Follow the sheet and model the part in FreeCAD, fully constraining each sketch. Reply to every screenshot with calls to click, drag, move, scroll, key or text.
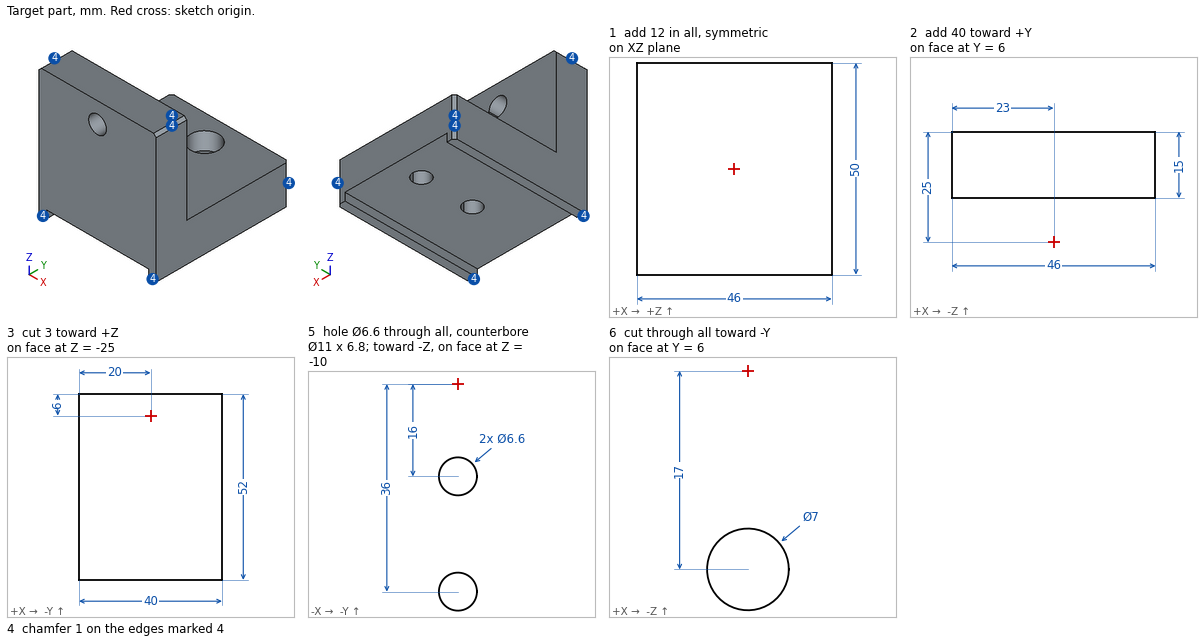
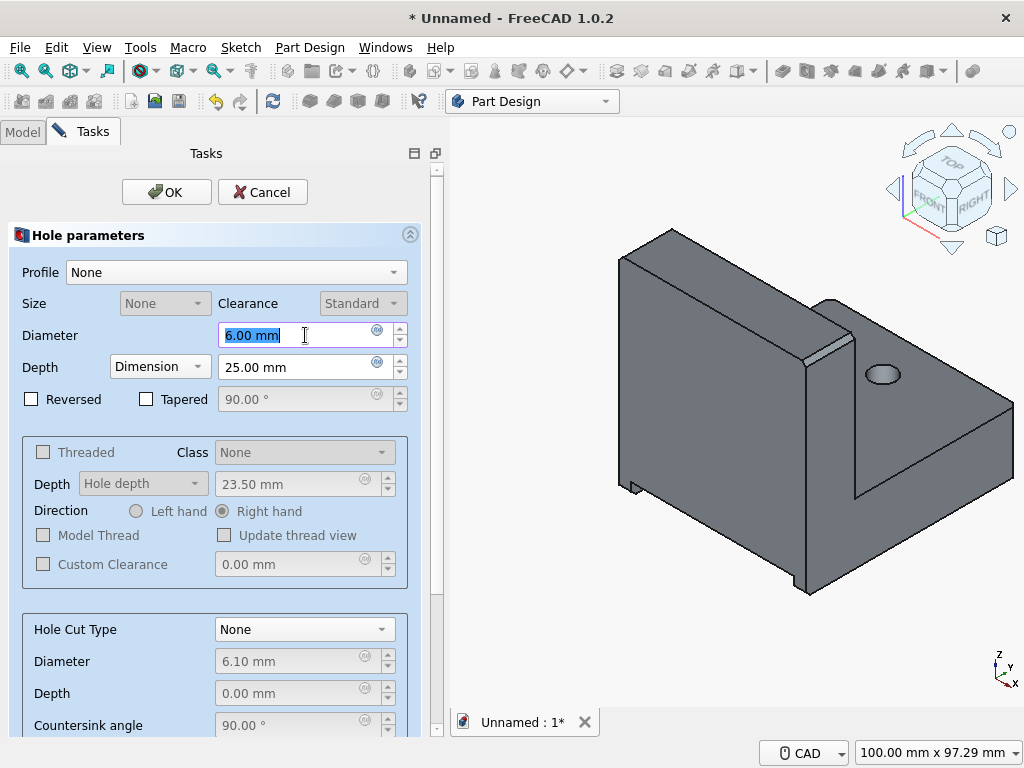
text(6.6)
key(Tab)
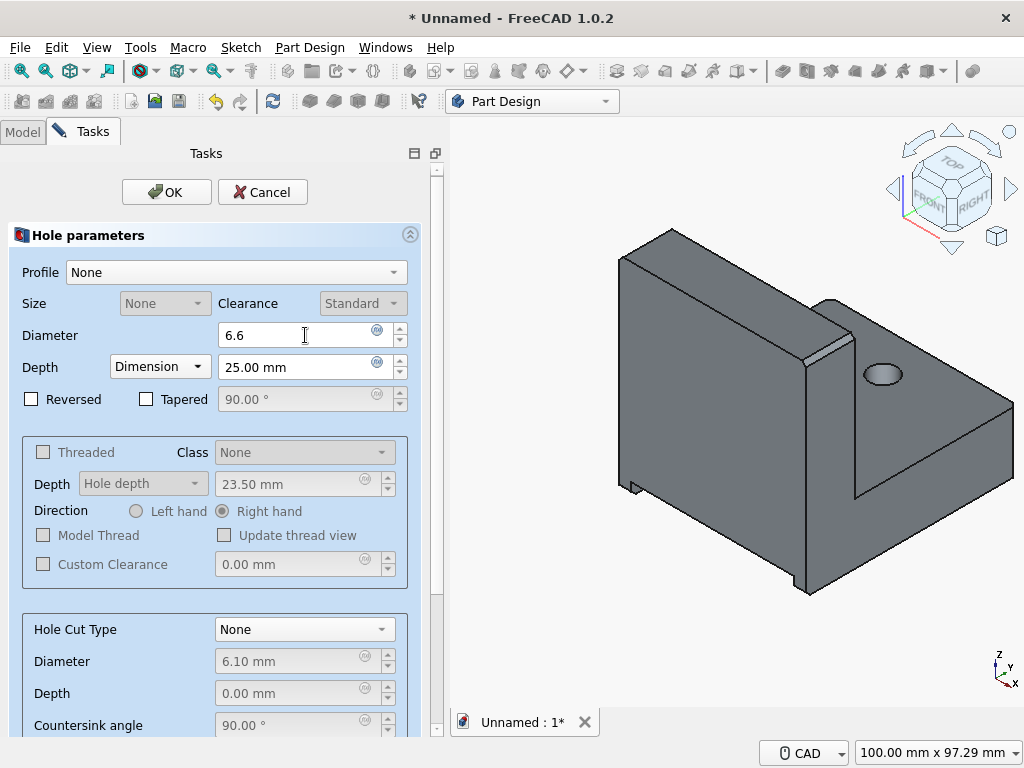
click(161, 366)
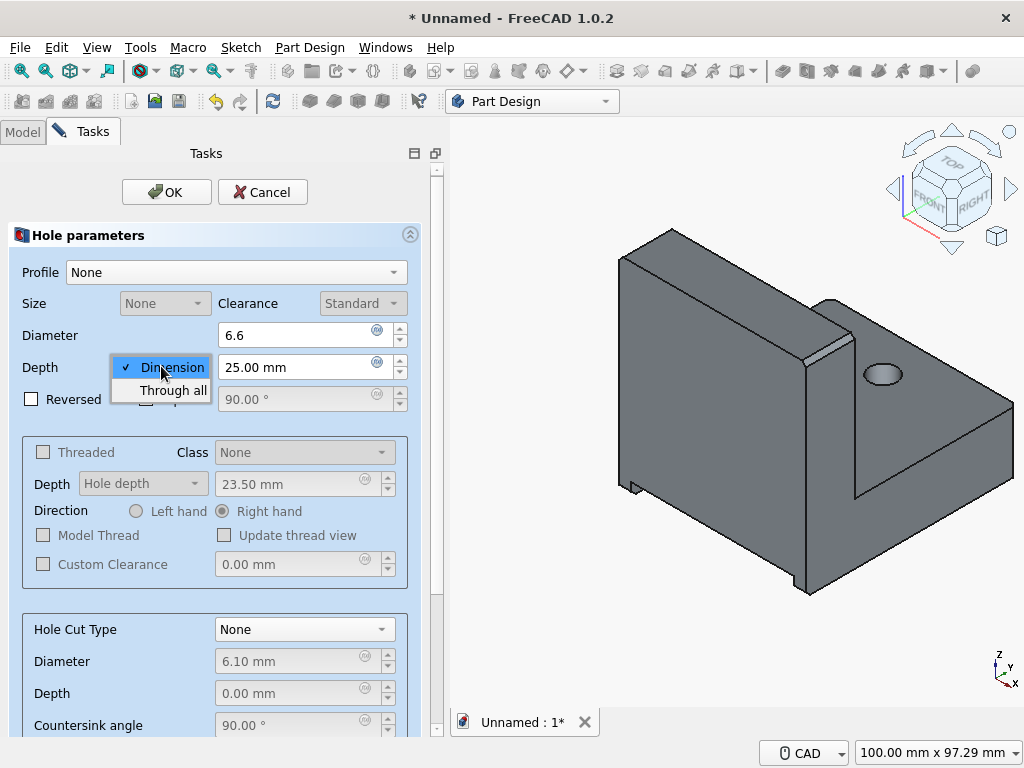
click(160, 390)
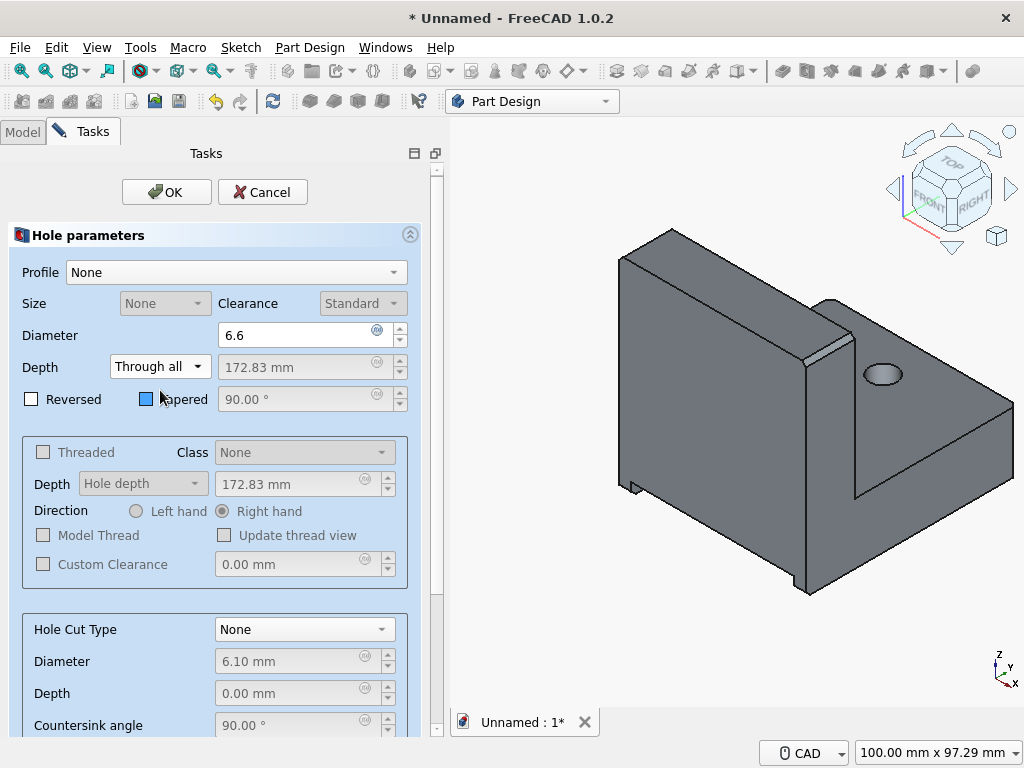
click(306, 630)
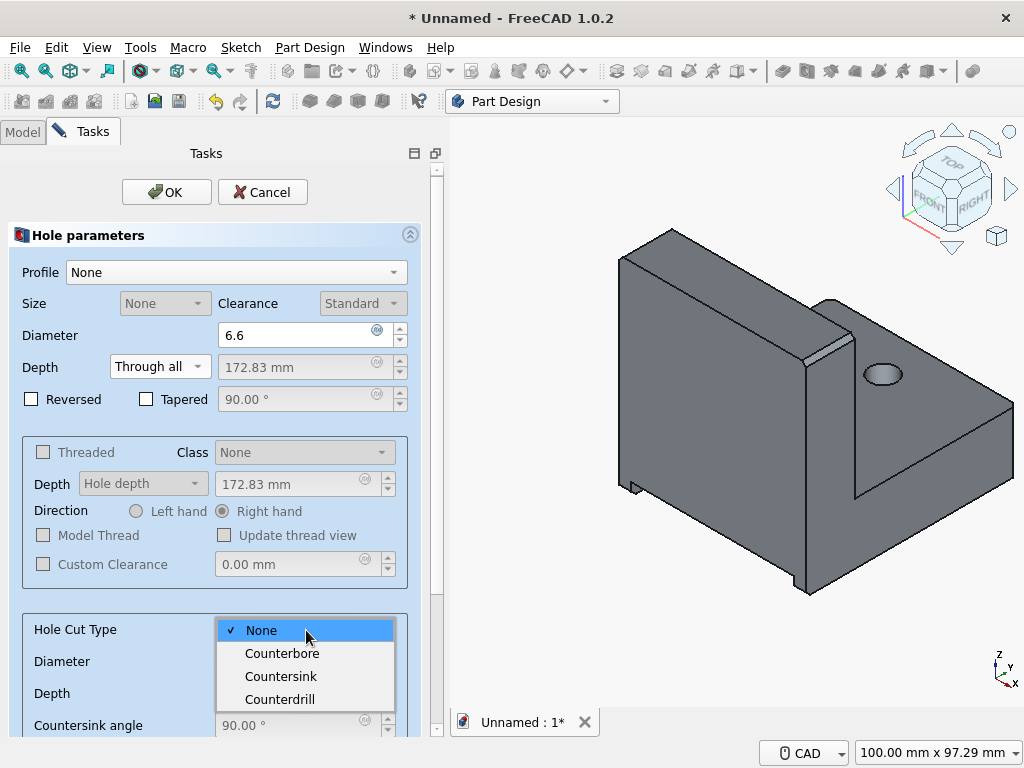
click(304, 654)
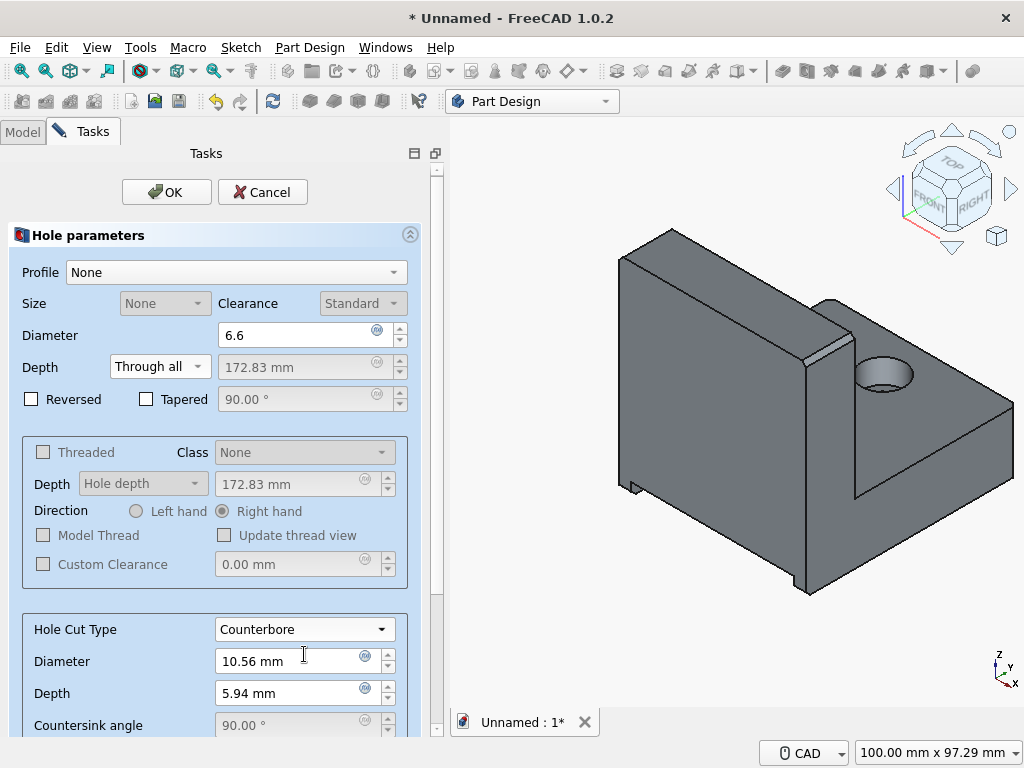
triple_click(298, 661)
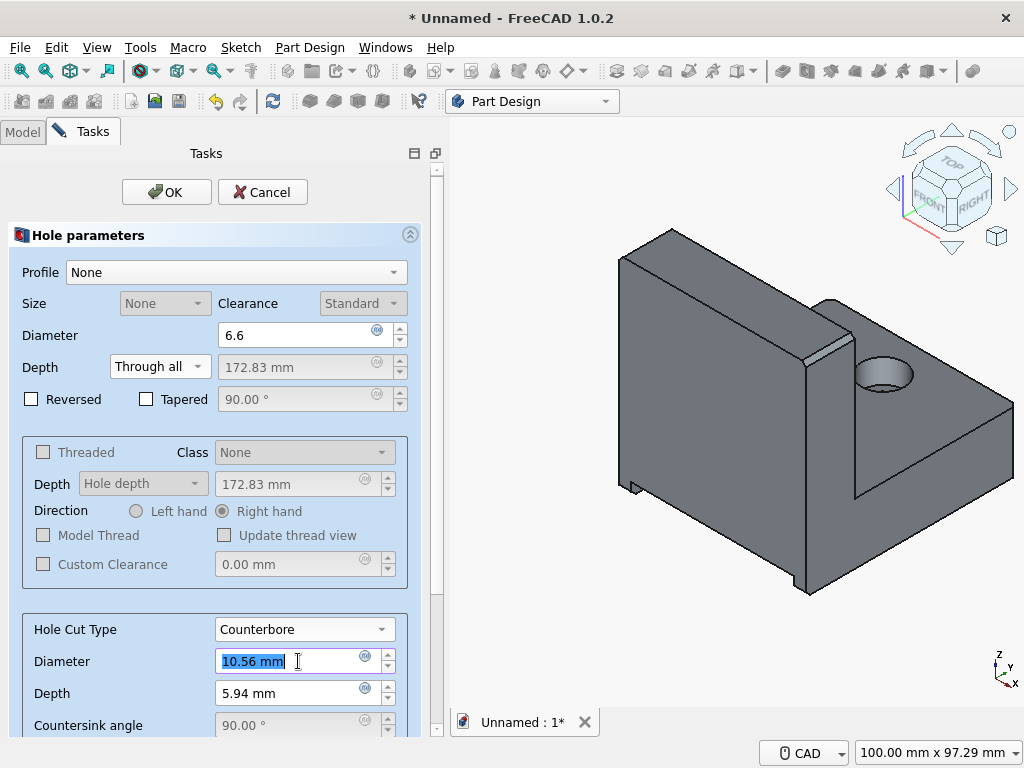
text(11)
key(Tab)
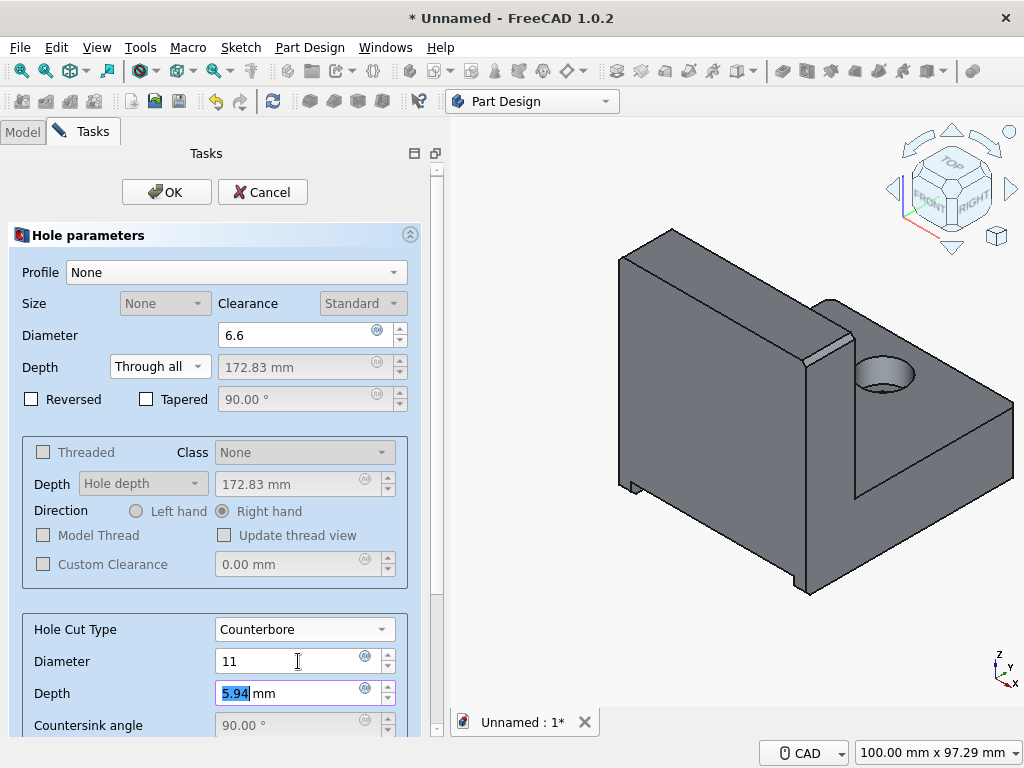
text(6.8)
key(Tab)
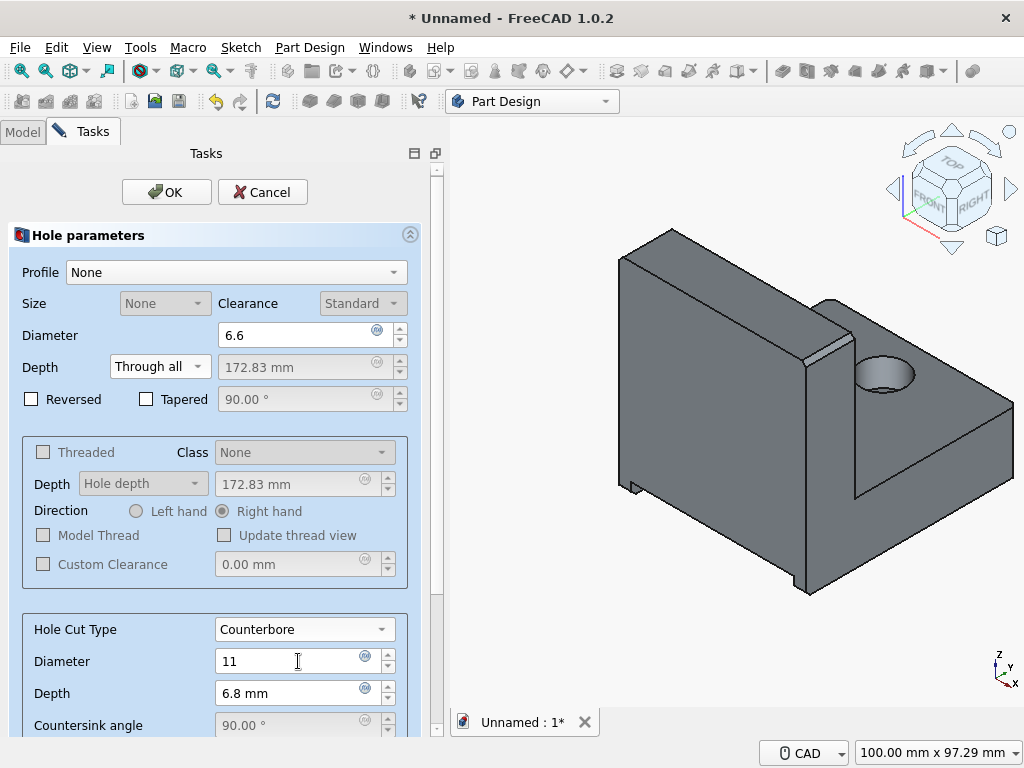
click(167, 192)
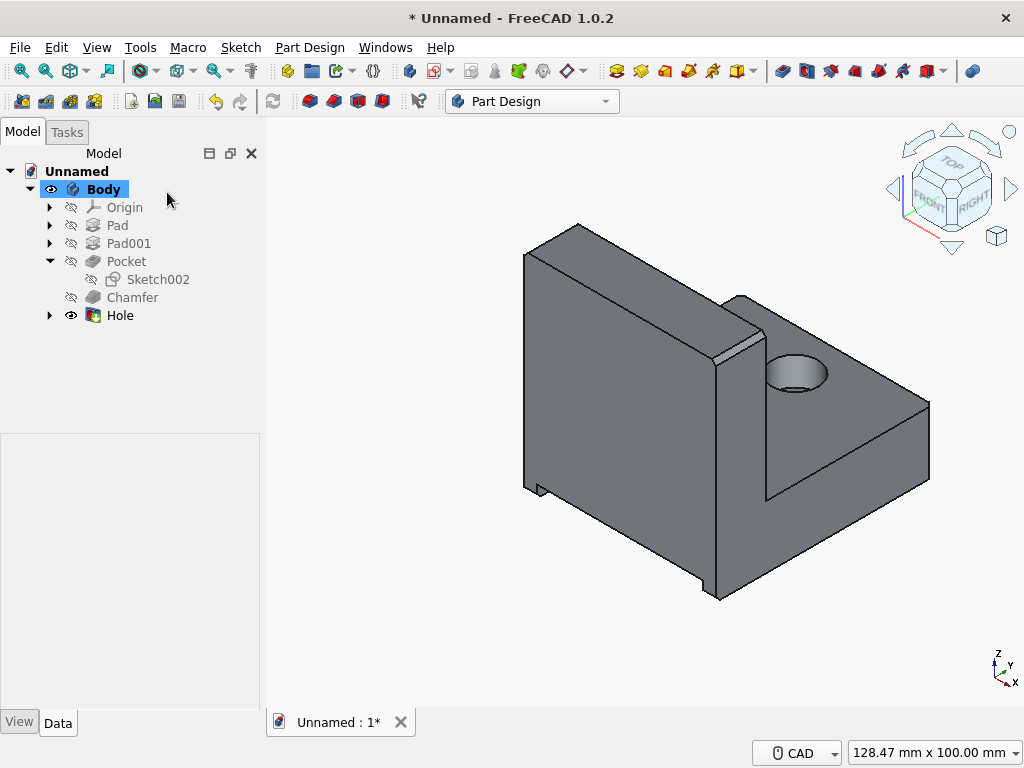
key(4)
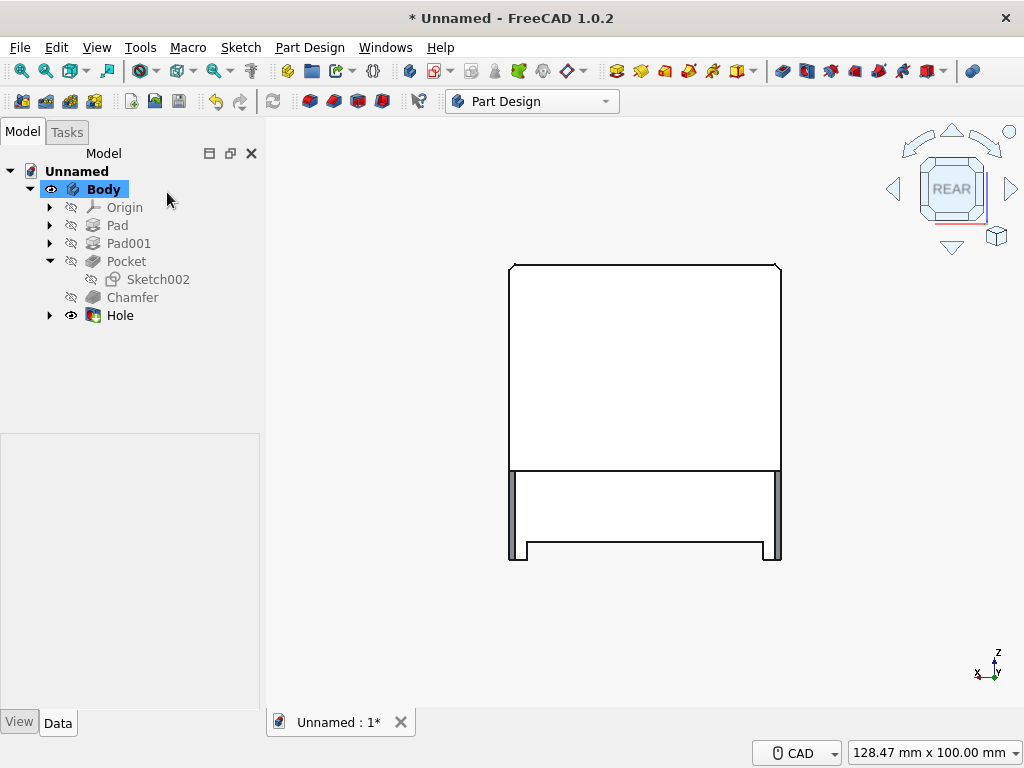
click(645, 367)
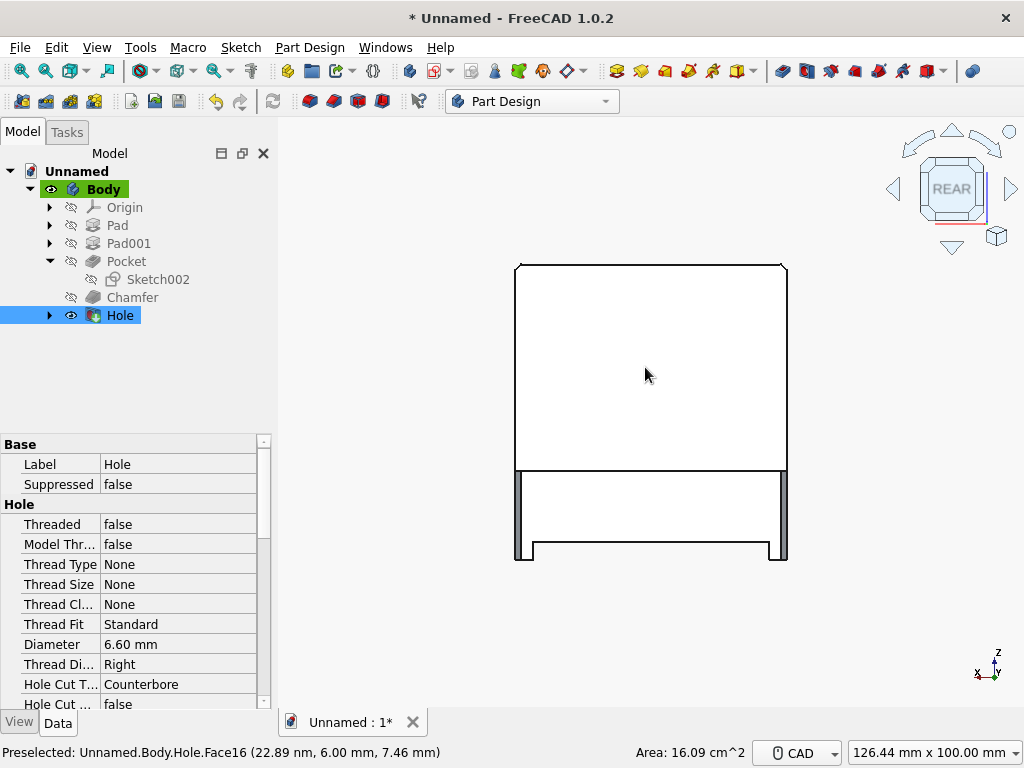
click(434, 72)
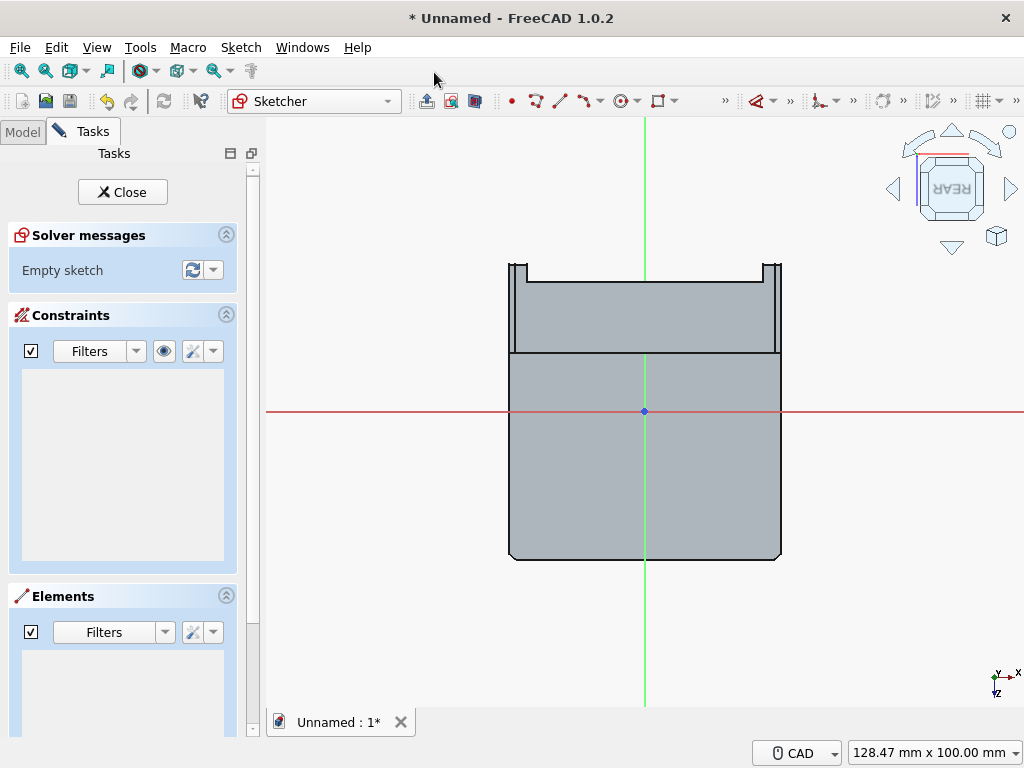
scroll(654, 525, up, 11)